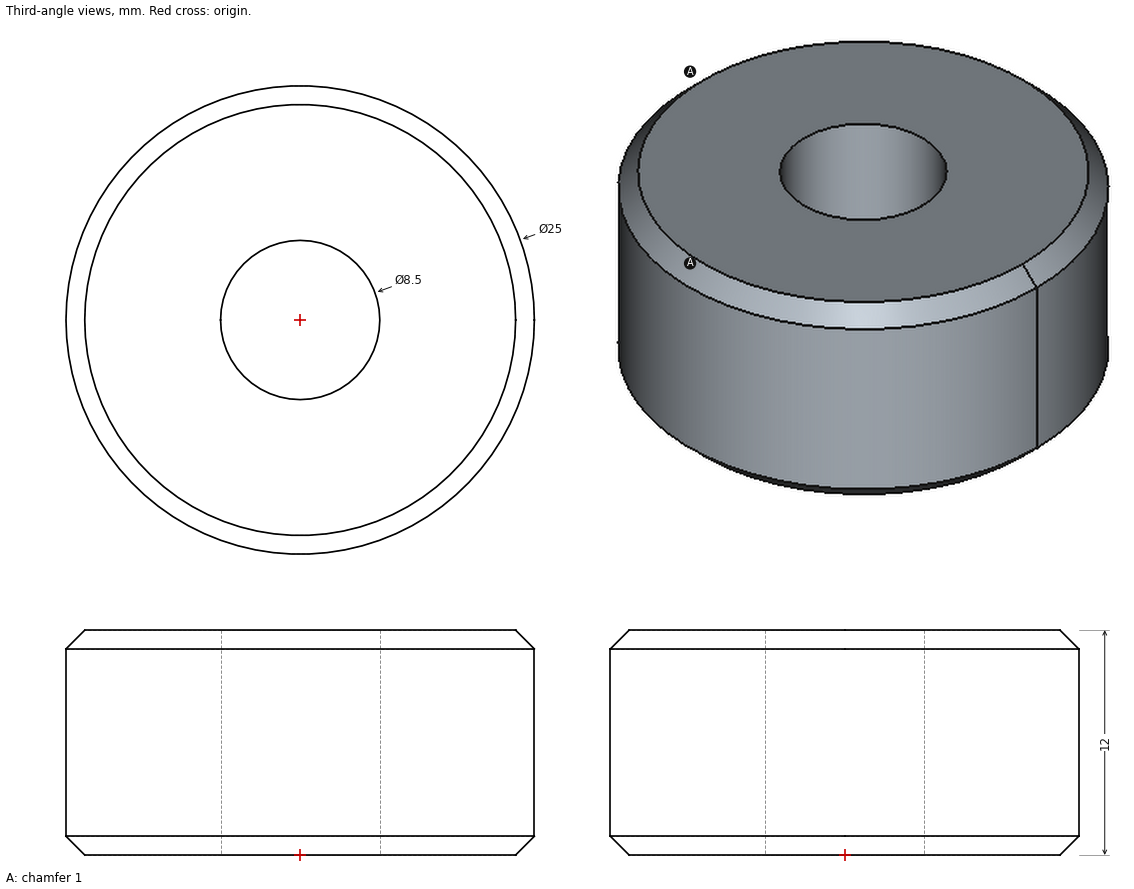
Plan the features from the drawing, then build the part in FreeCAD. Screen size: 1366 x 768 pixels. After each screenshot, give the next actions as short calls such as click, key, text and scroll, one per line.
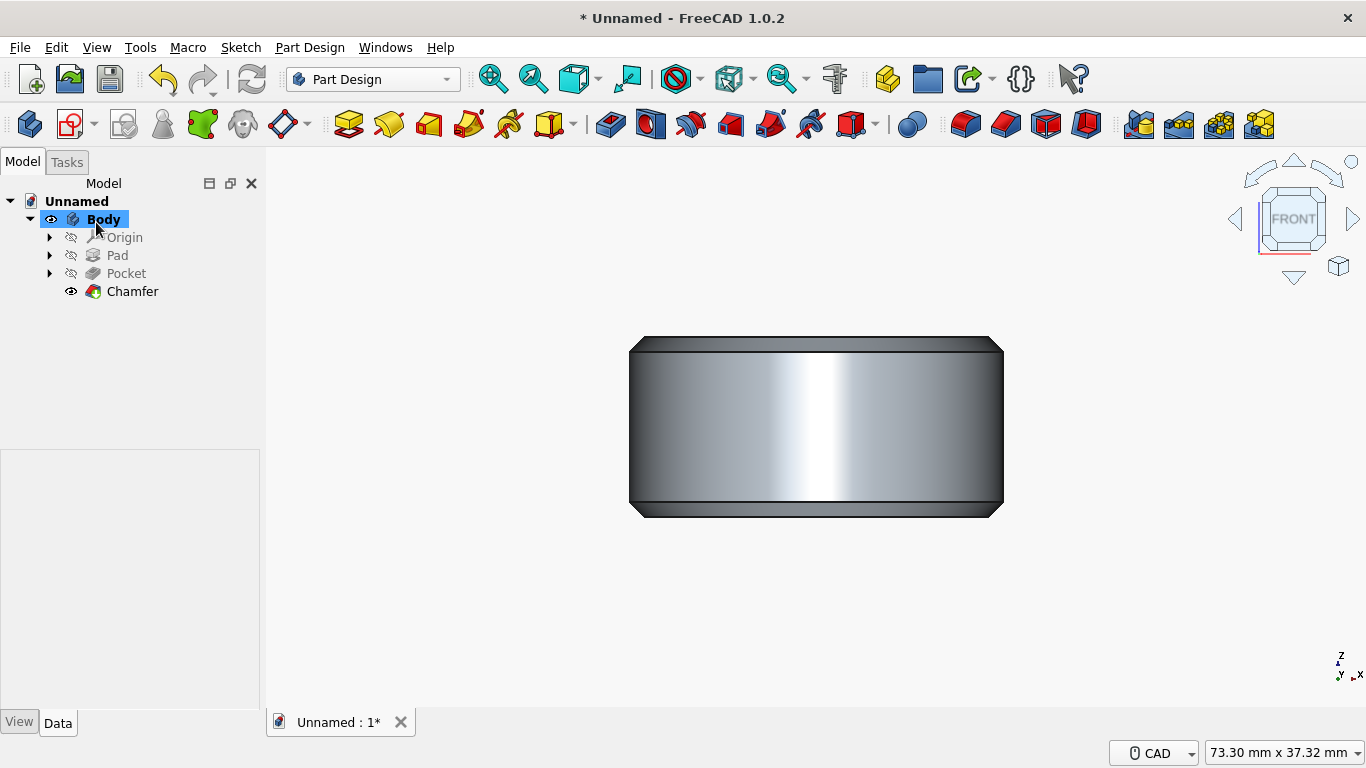
key(0)